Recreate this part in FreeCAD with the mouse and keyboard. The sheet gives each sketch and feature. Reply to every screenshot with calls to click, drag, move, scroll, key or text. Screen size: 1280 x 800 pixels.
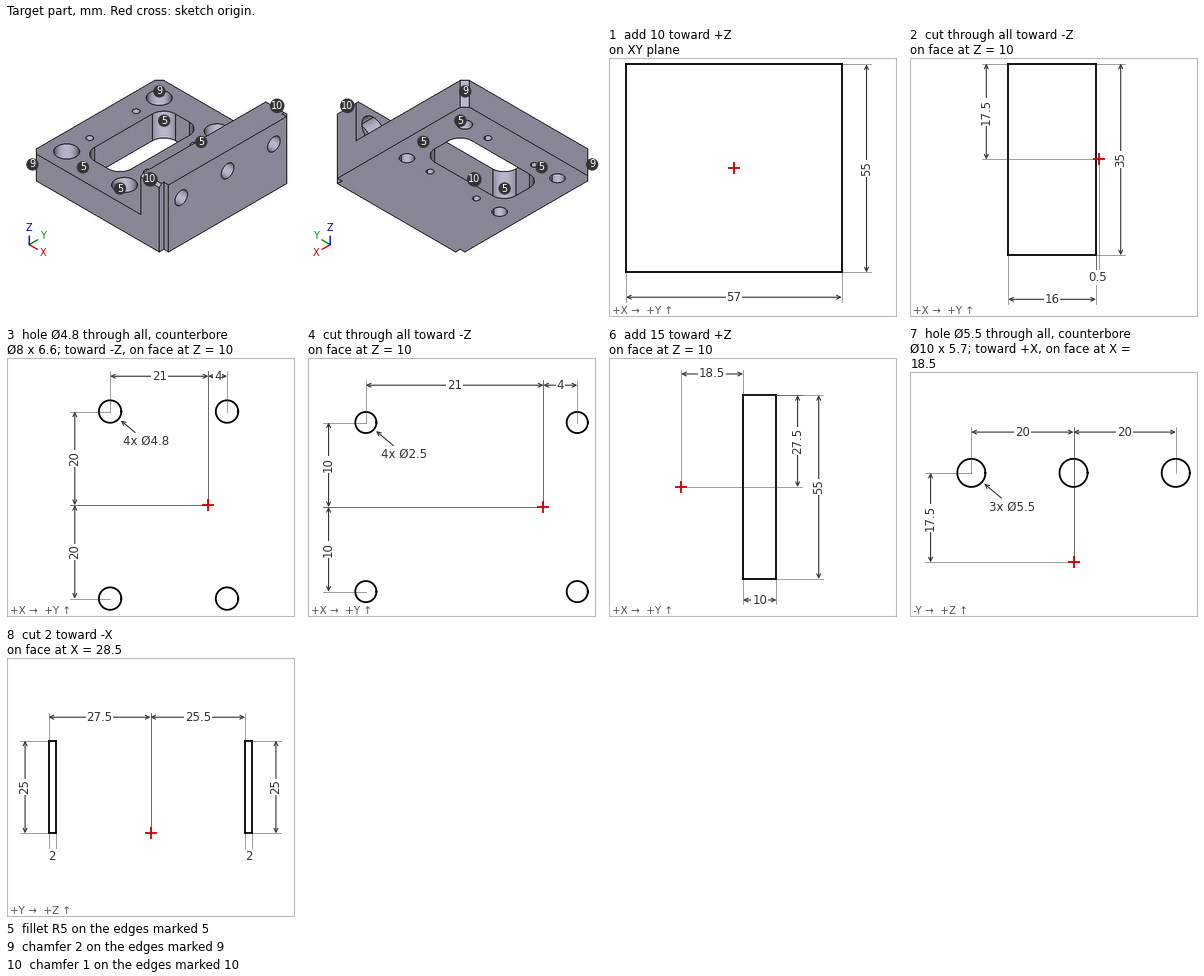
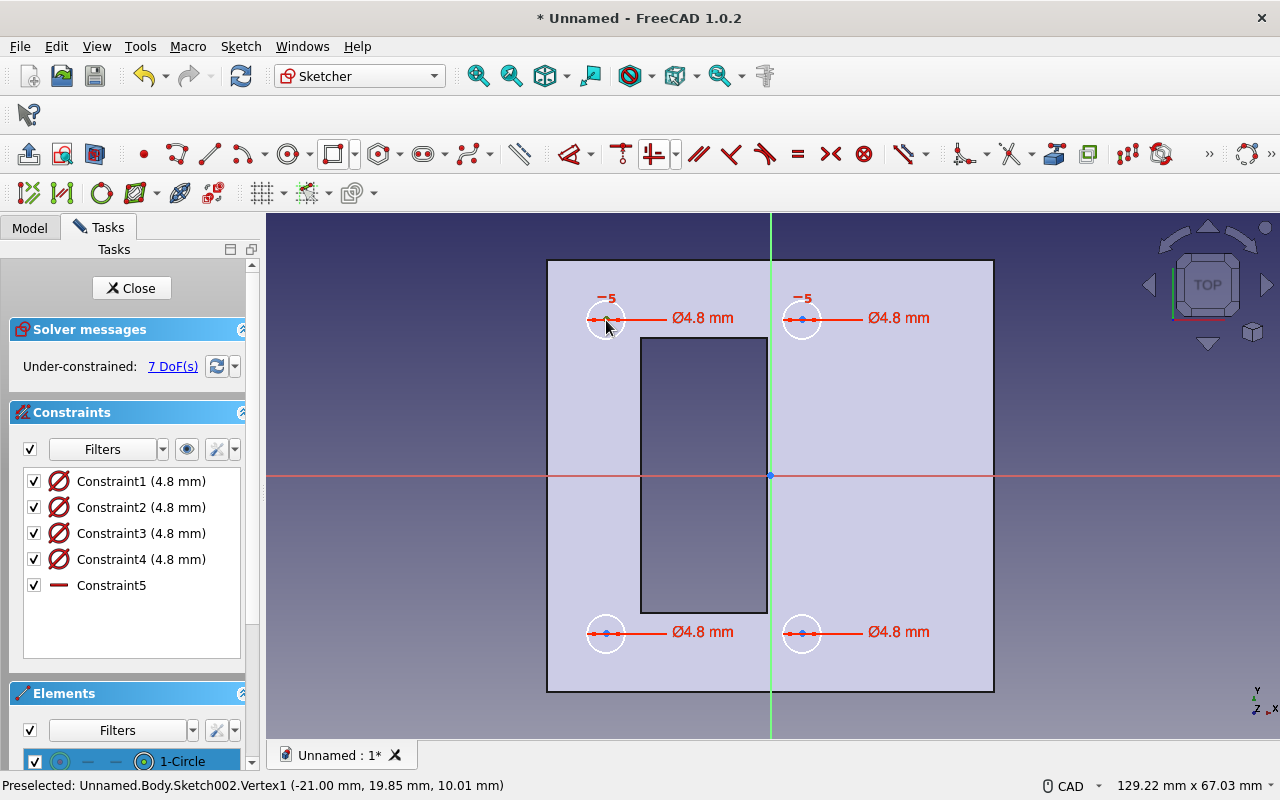
click(606, 634)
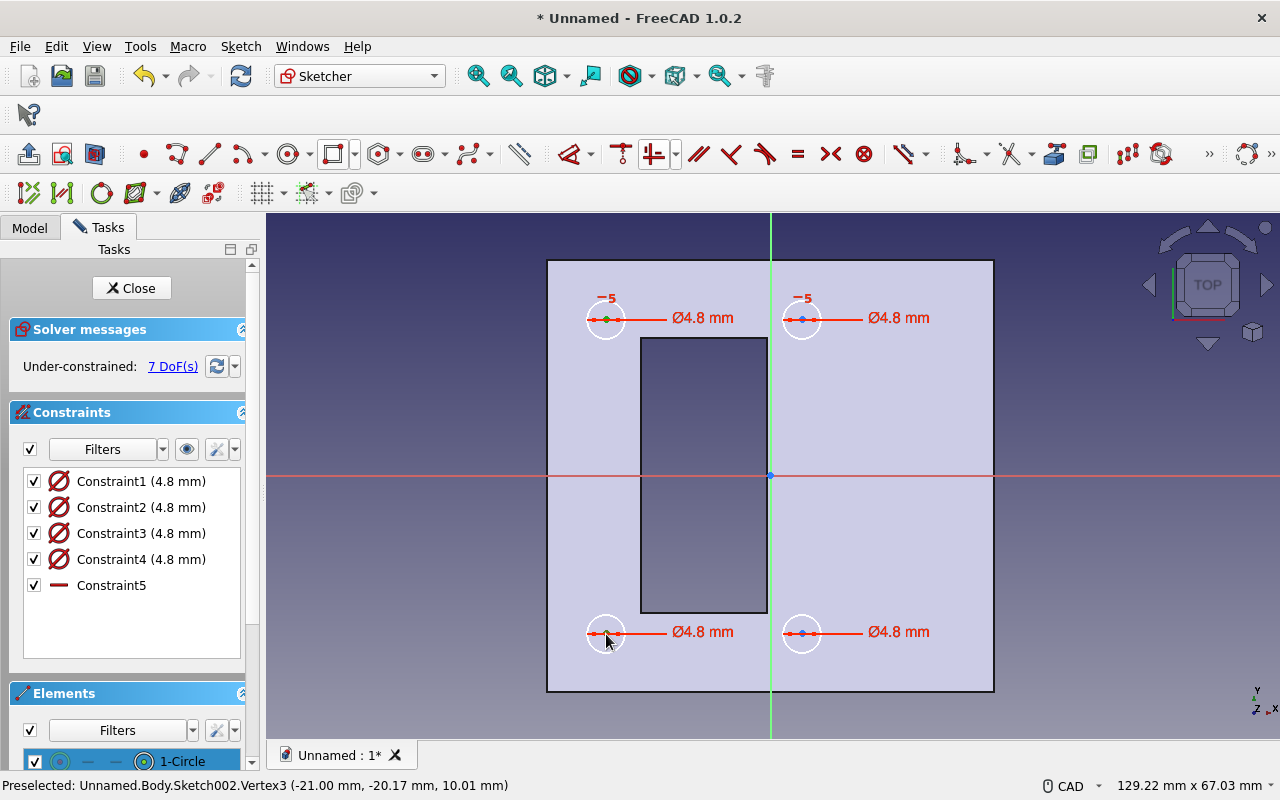
click(676, 154)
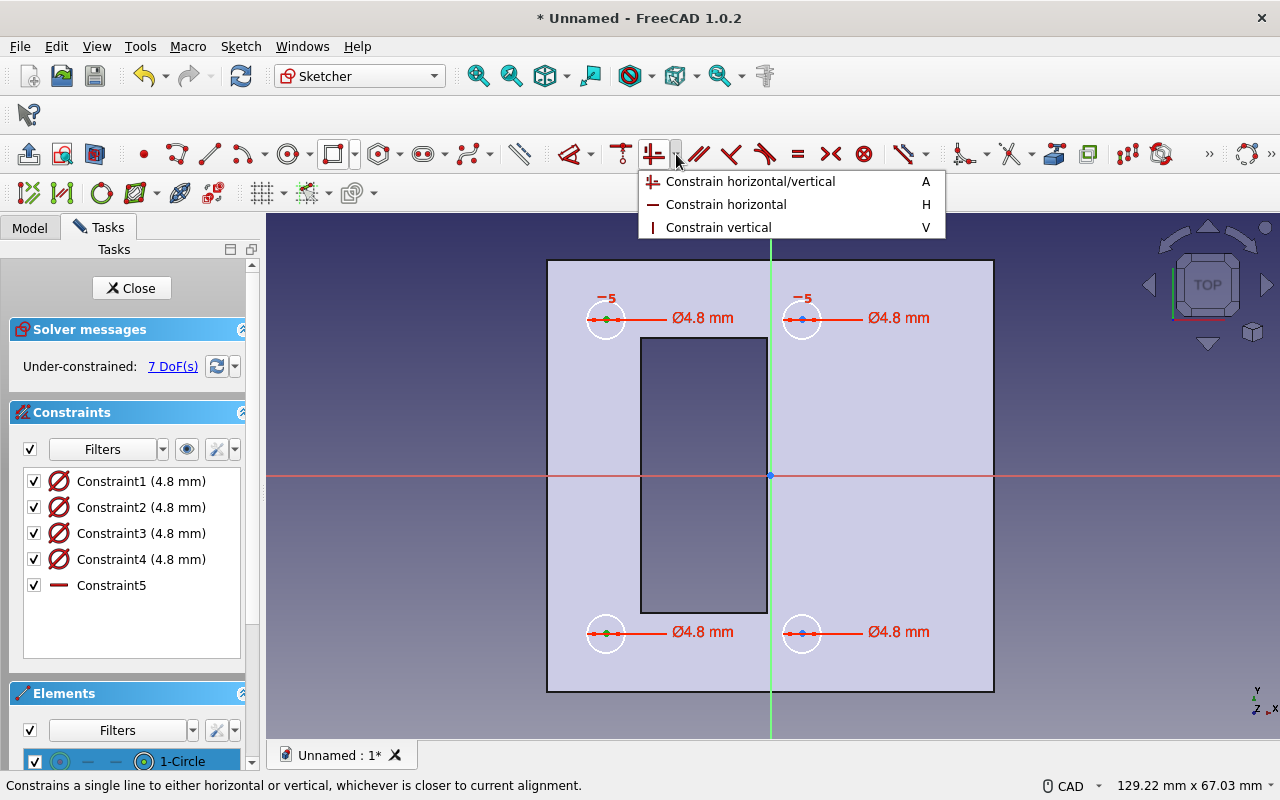
click(792, 228)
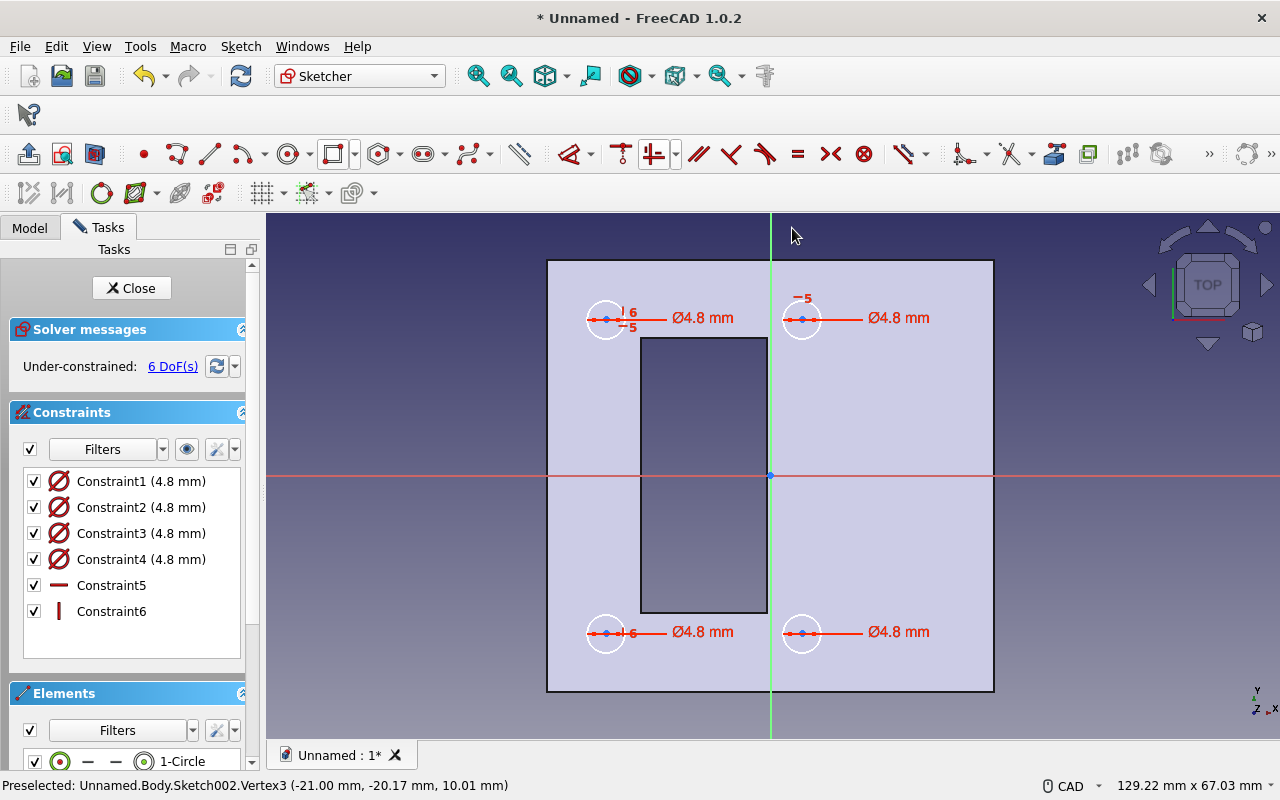
click(802, 320)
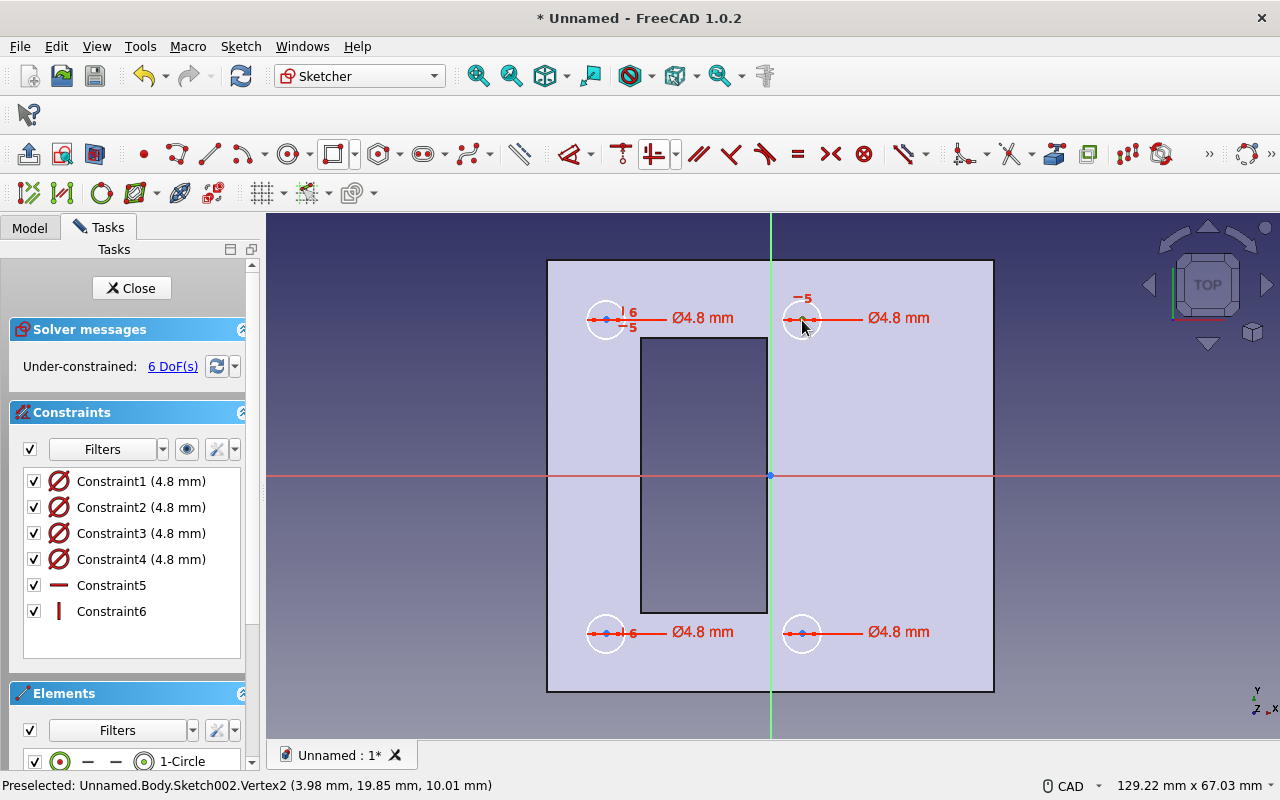
click(802, 634)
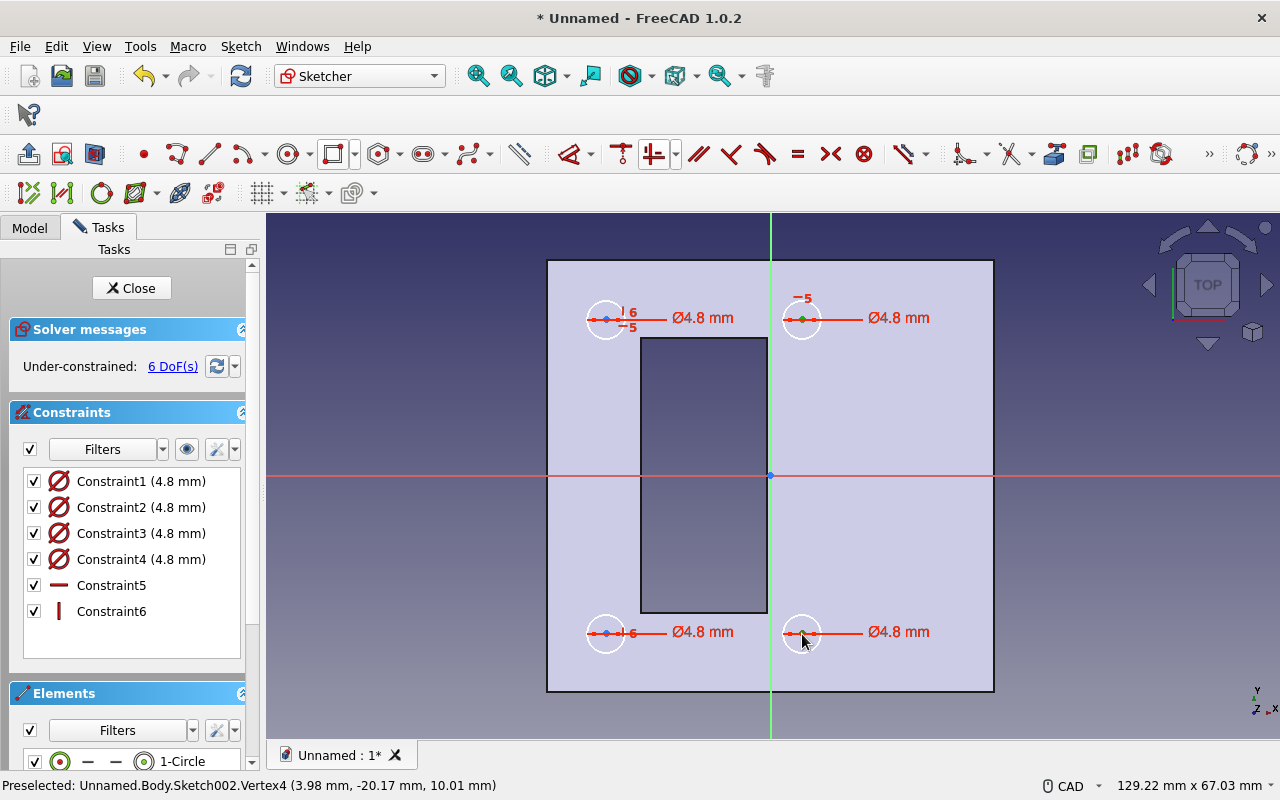
key(v)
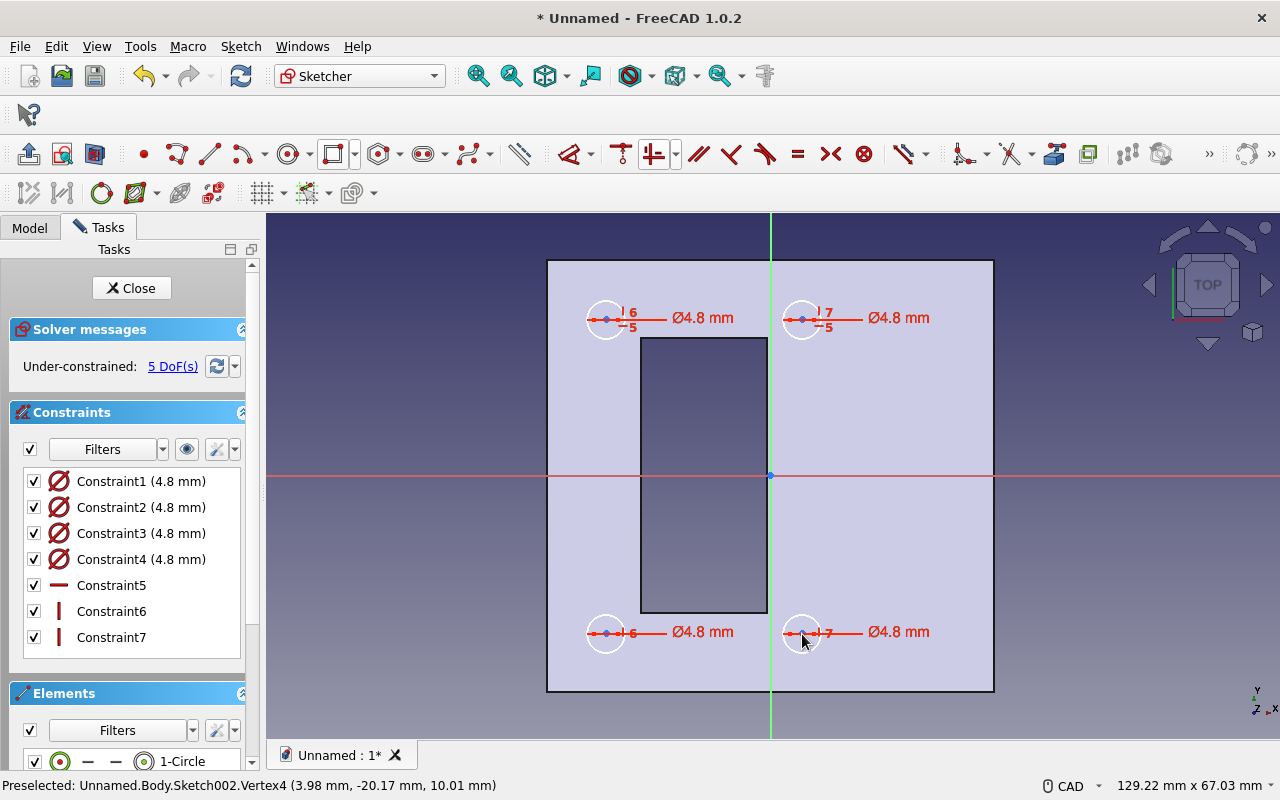
click(606, 634)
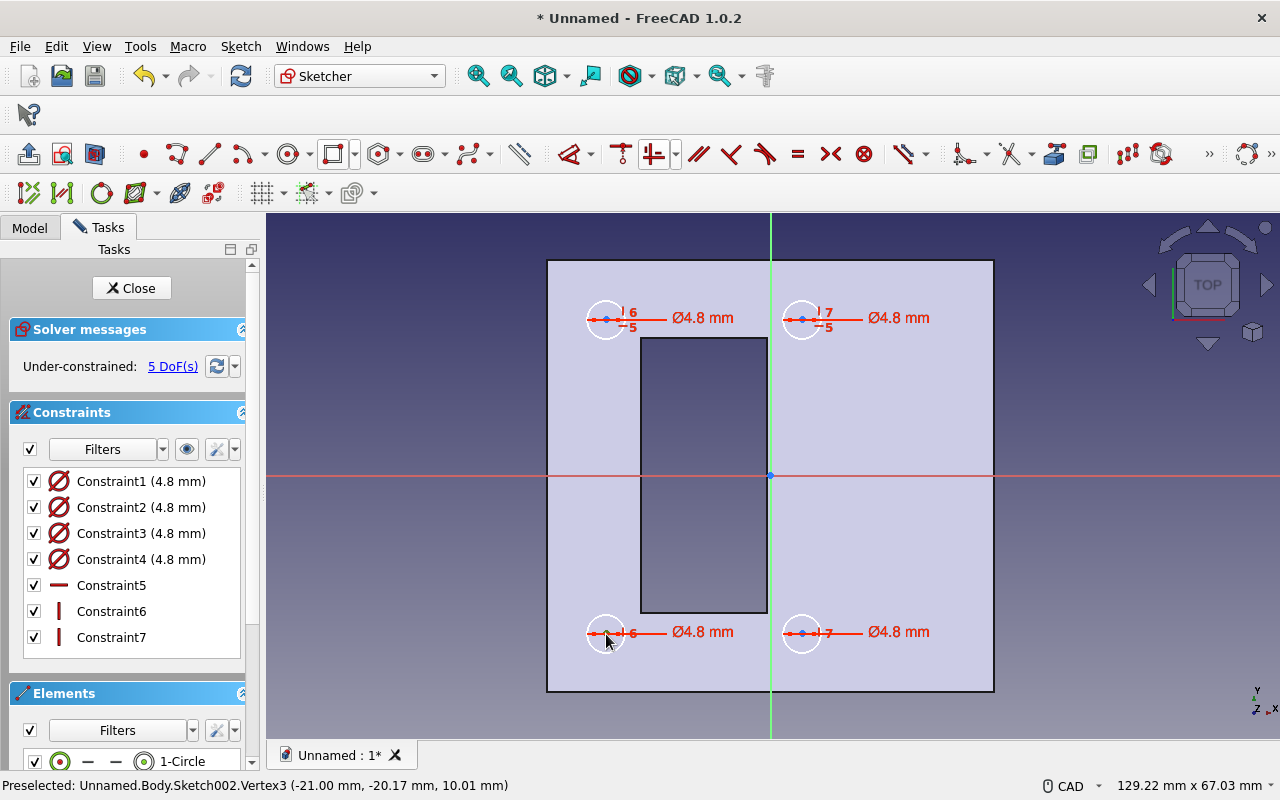
click(802, 634)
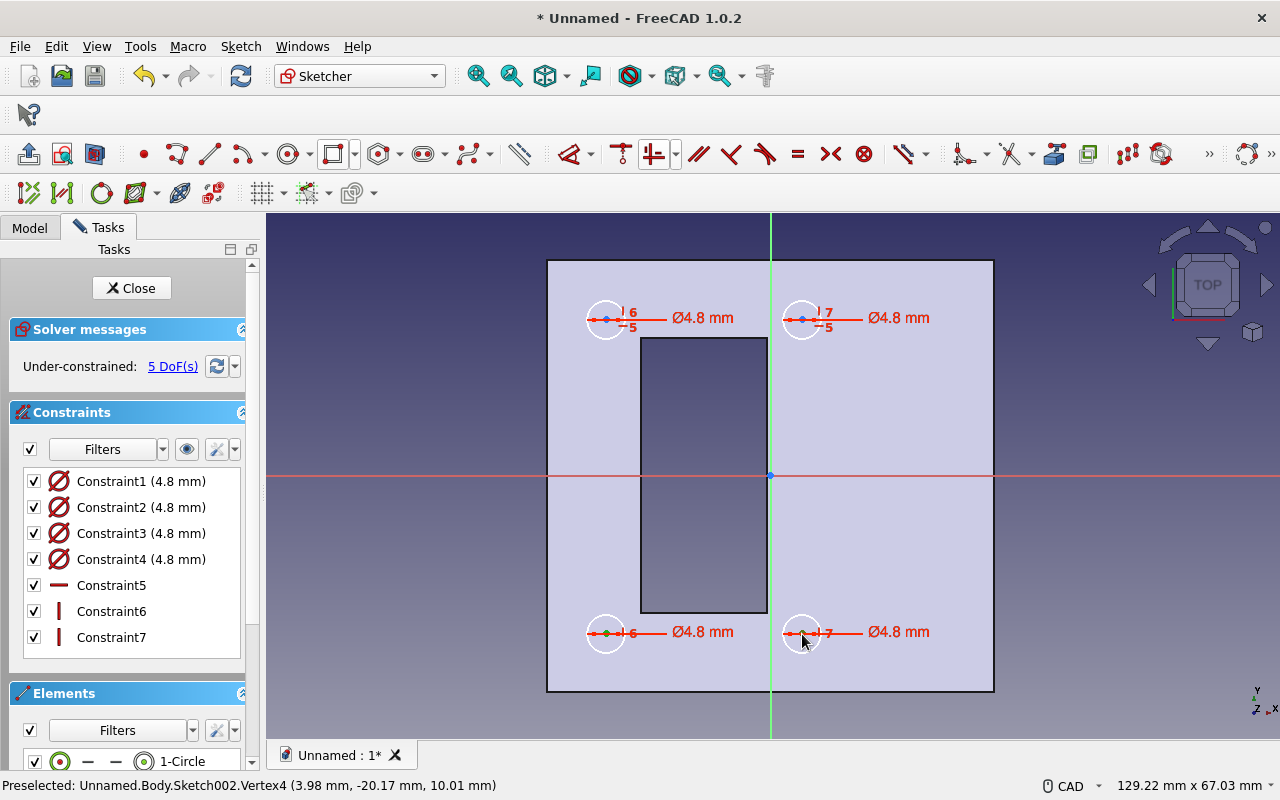
key(h)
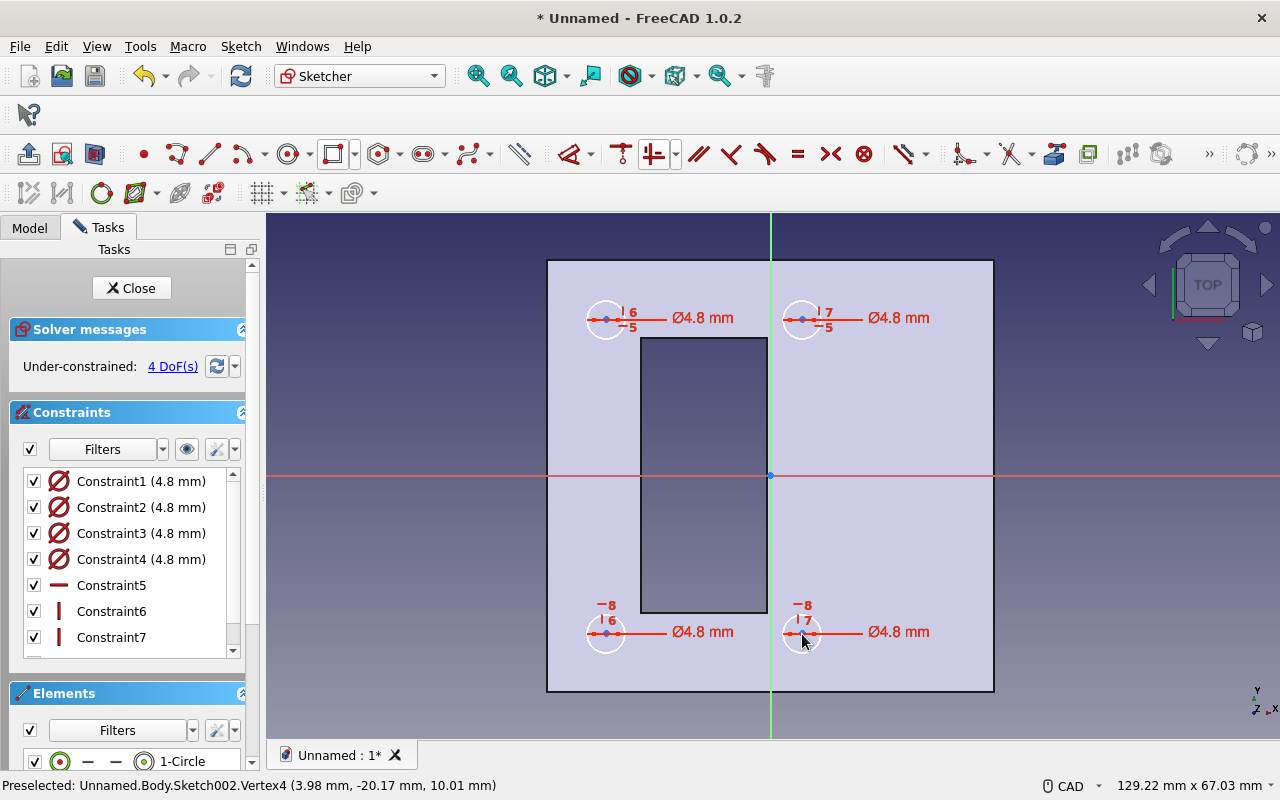
scroll(802, 320, up, 2)